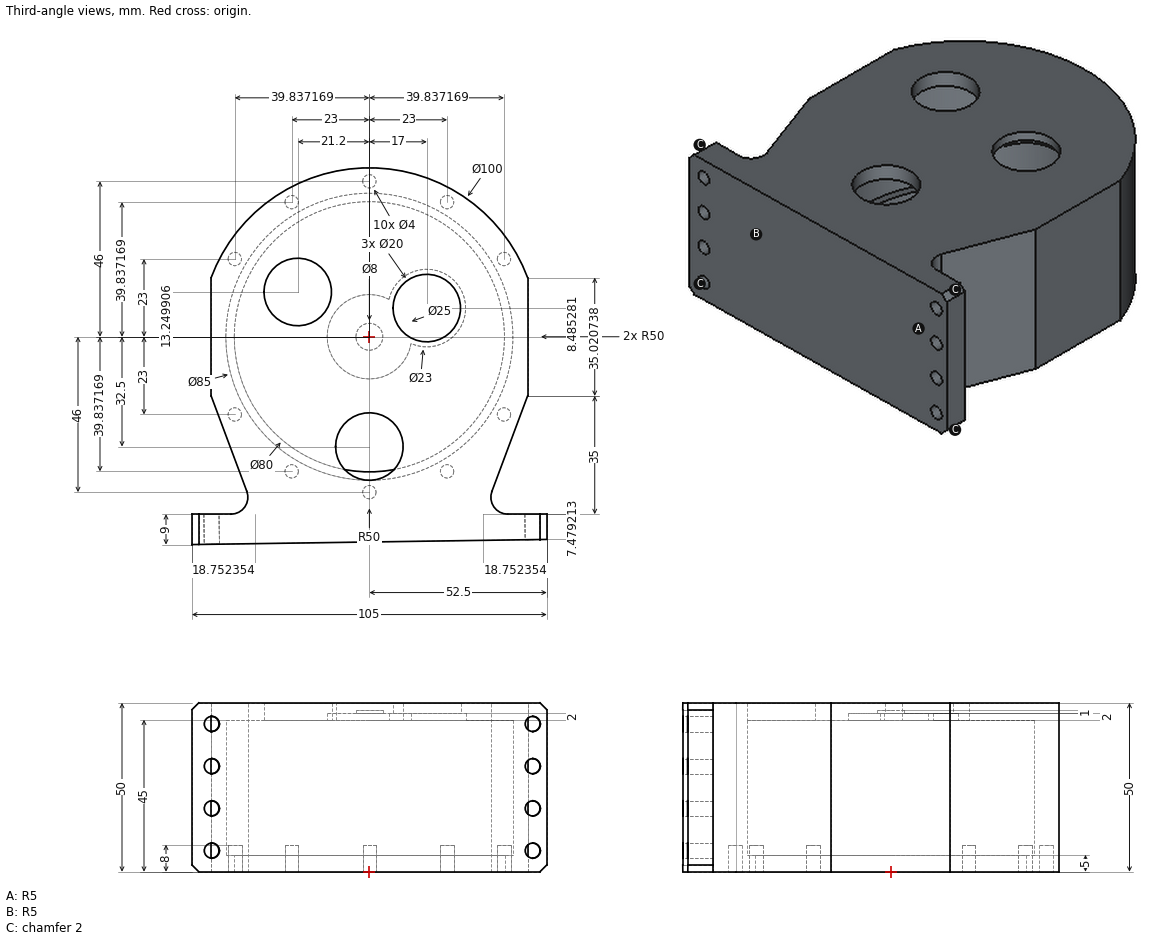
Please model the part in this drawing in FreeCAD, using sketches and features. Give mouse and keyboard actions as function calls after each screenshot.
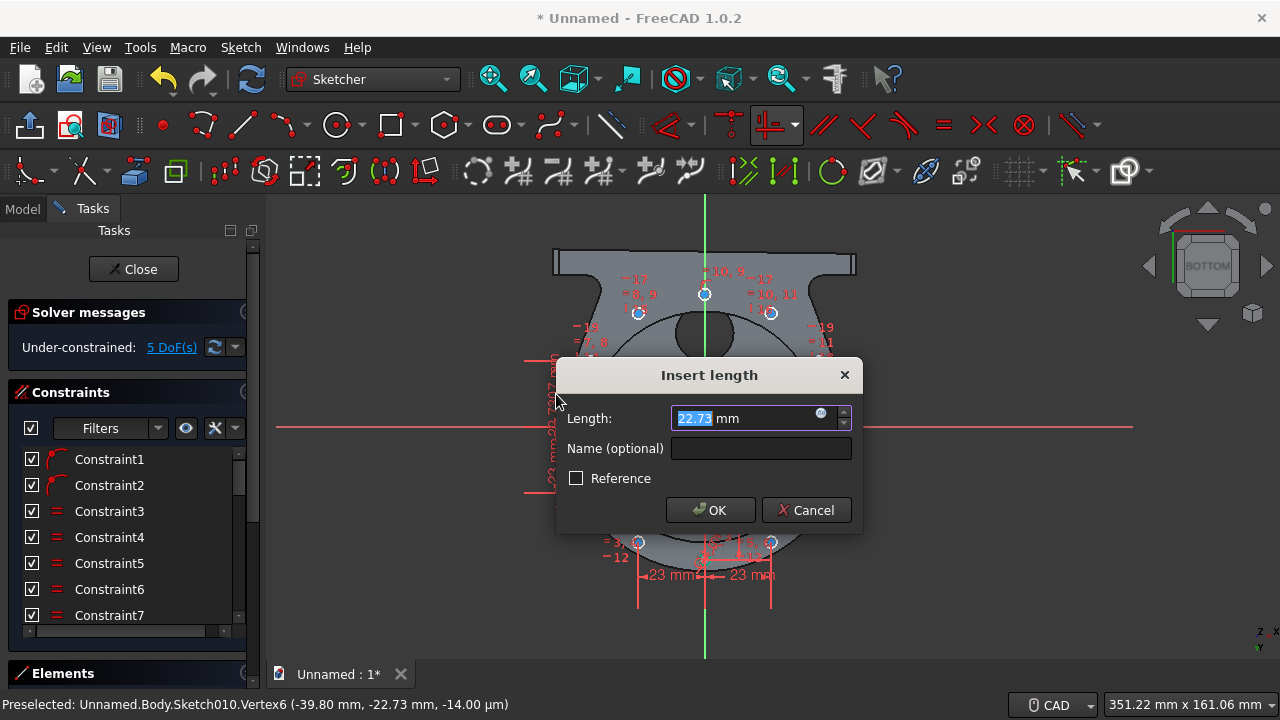
text(23)
key(Return)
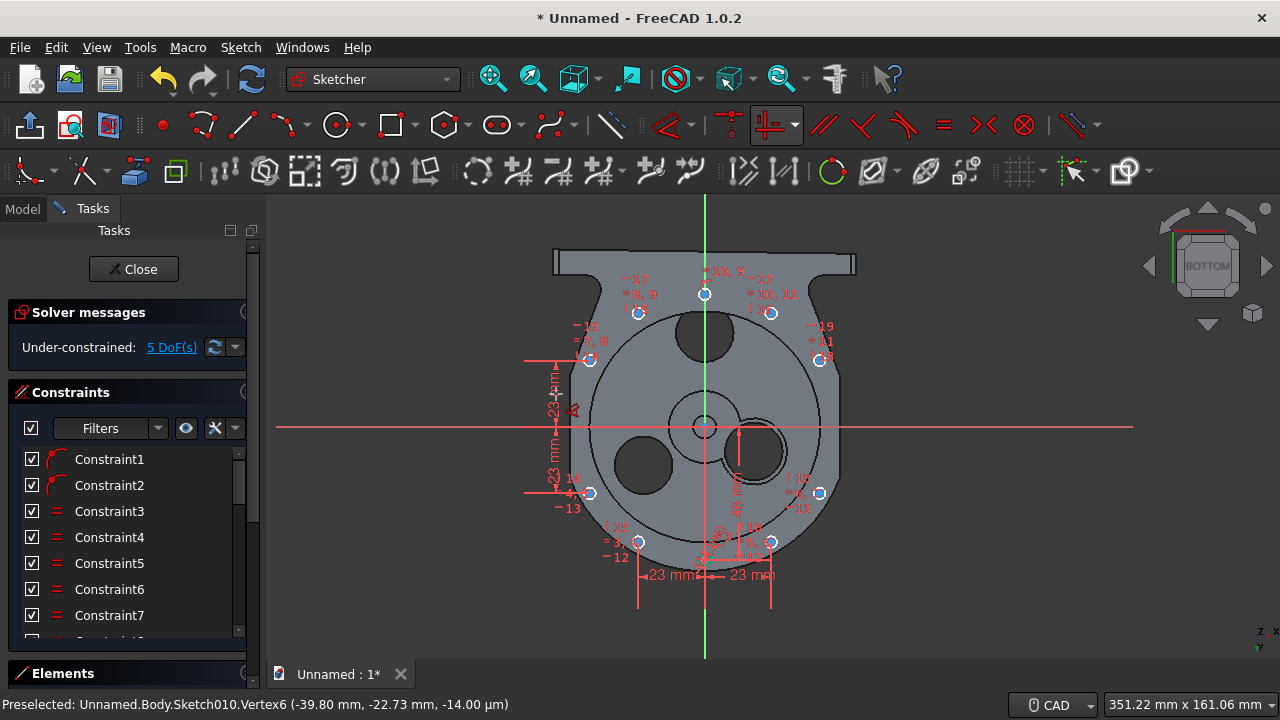
click(705, 294)
click(739, 361)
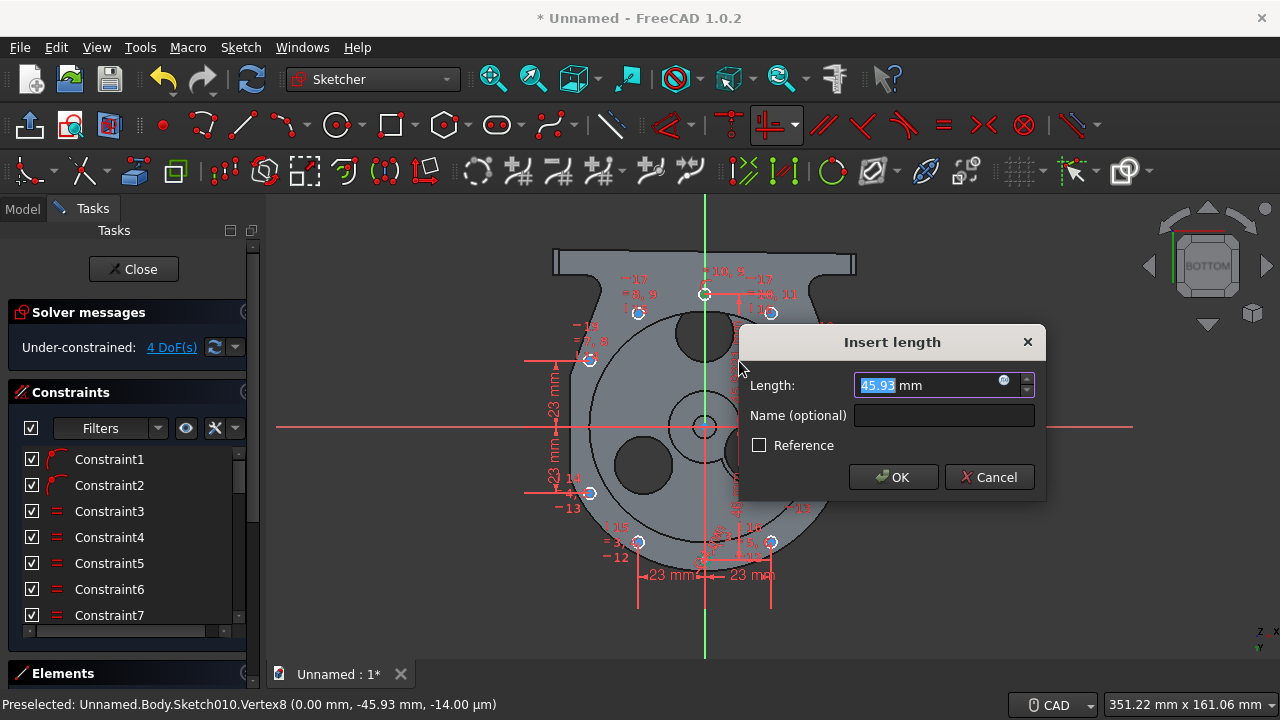
text(46)
key(Return)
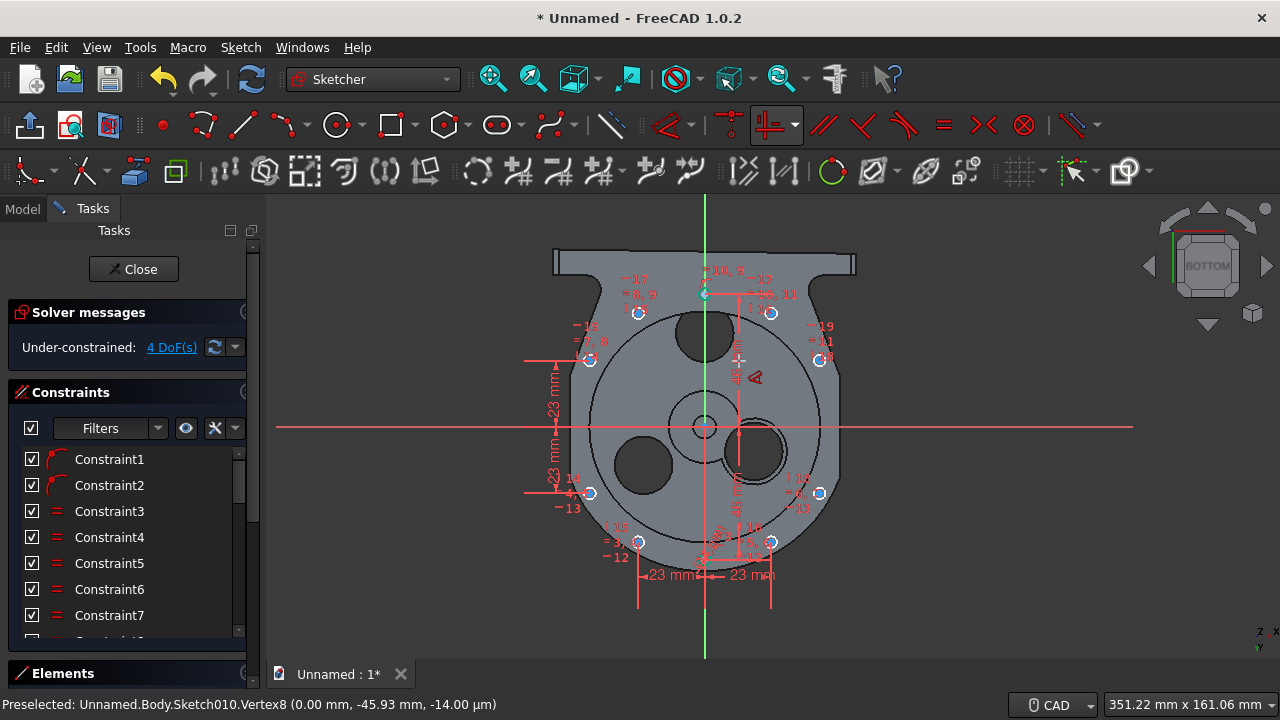
click(638, 542)
click(604, 511)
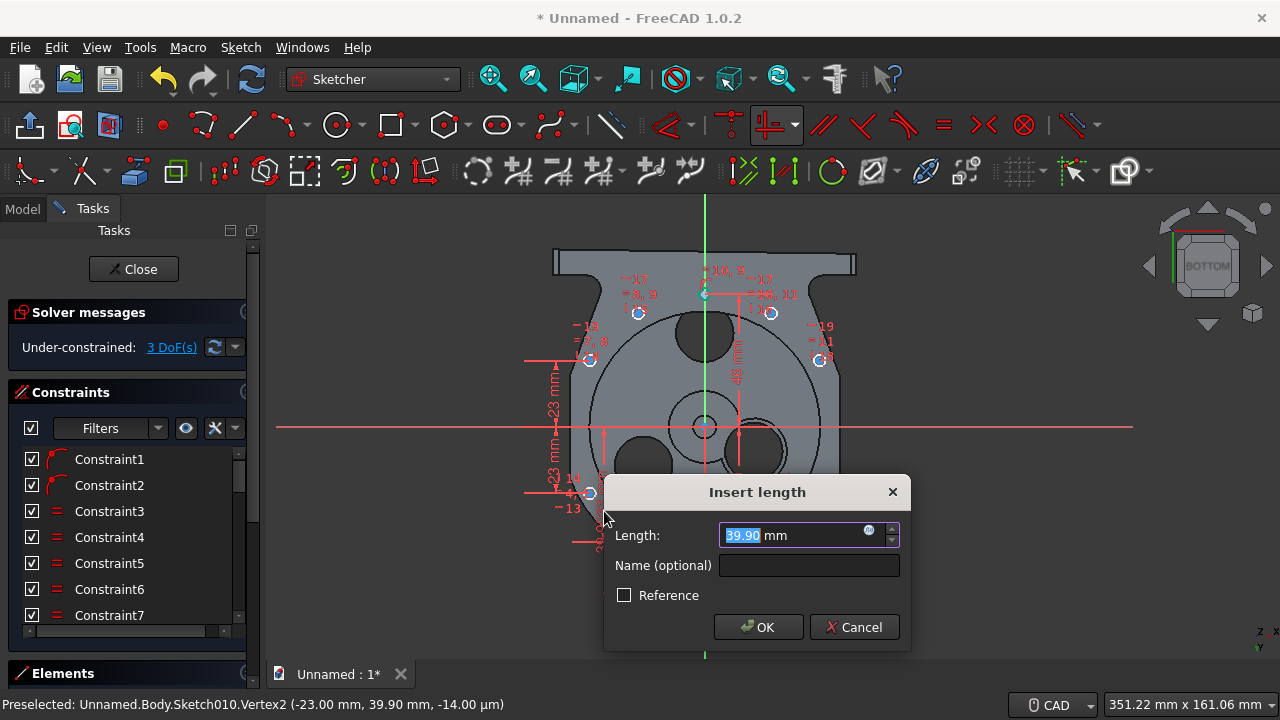
text(39.837169)
key(Return)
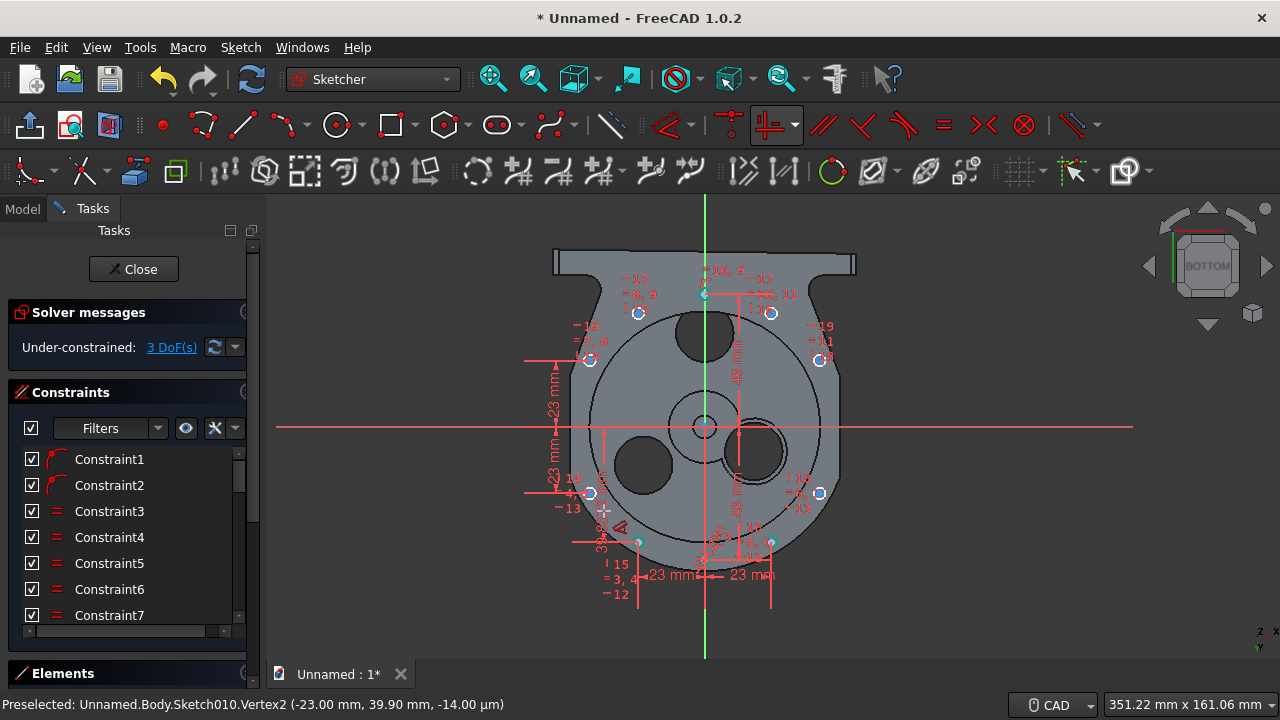
click(590, 493)
click(688, 527)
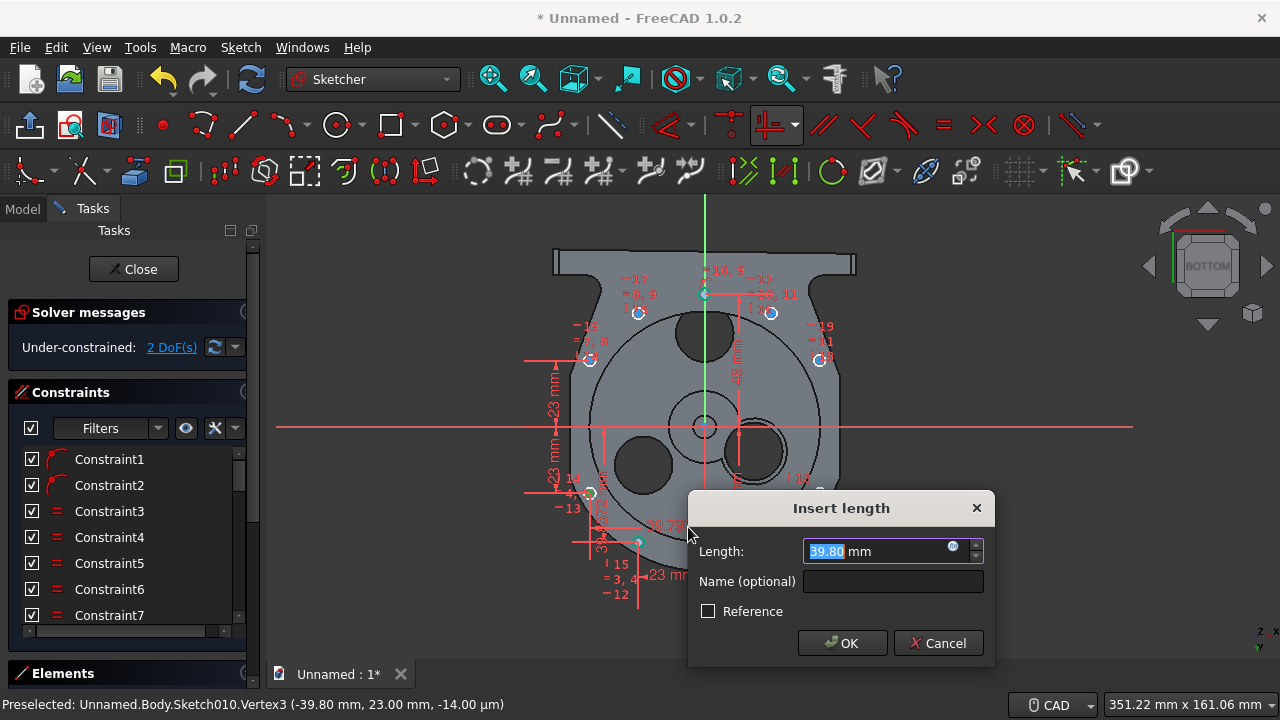
text(39.837169)
key(Return)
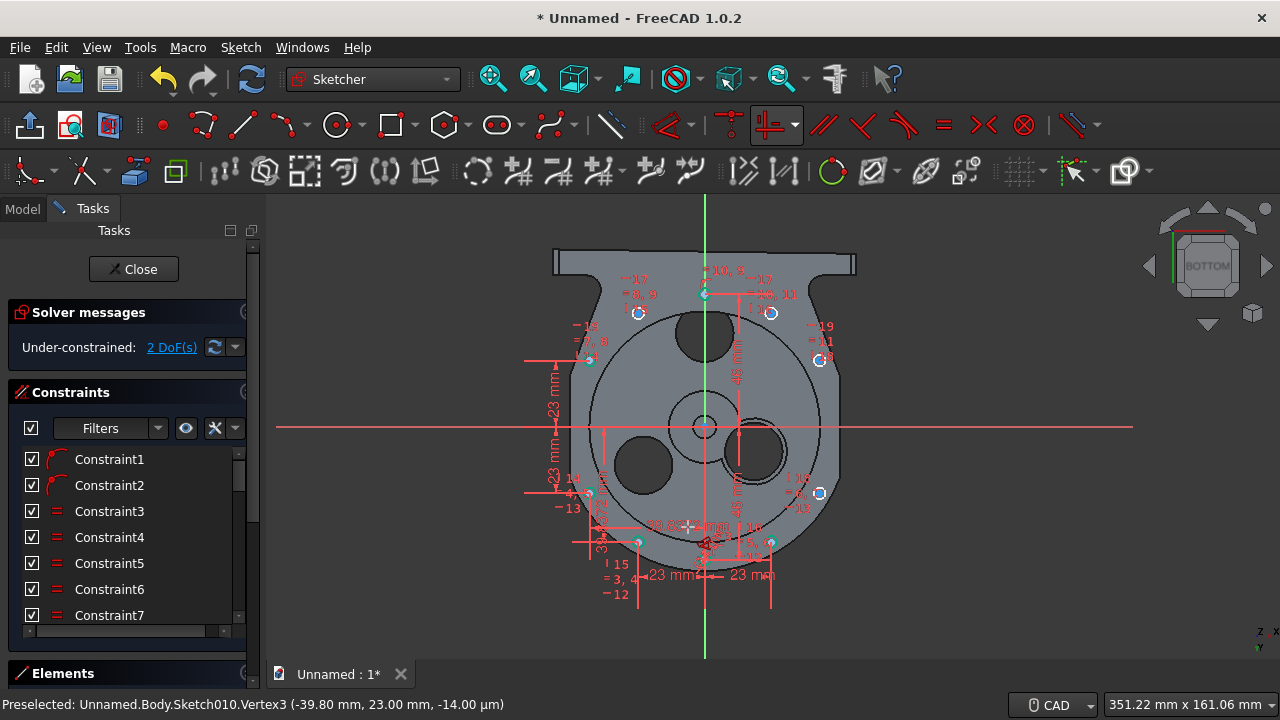
click(820, 493)
click(789, 527)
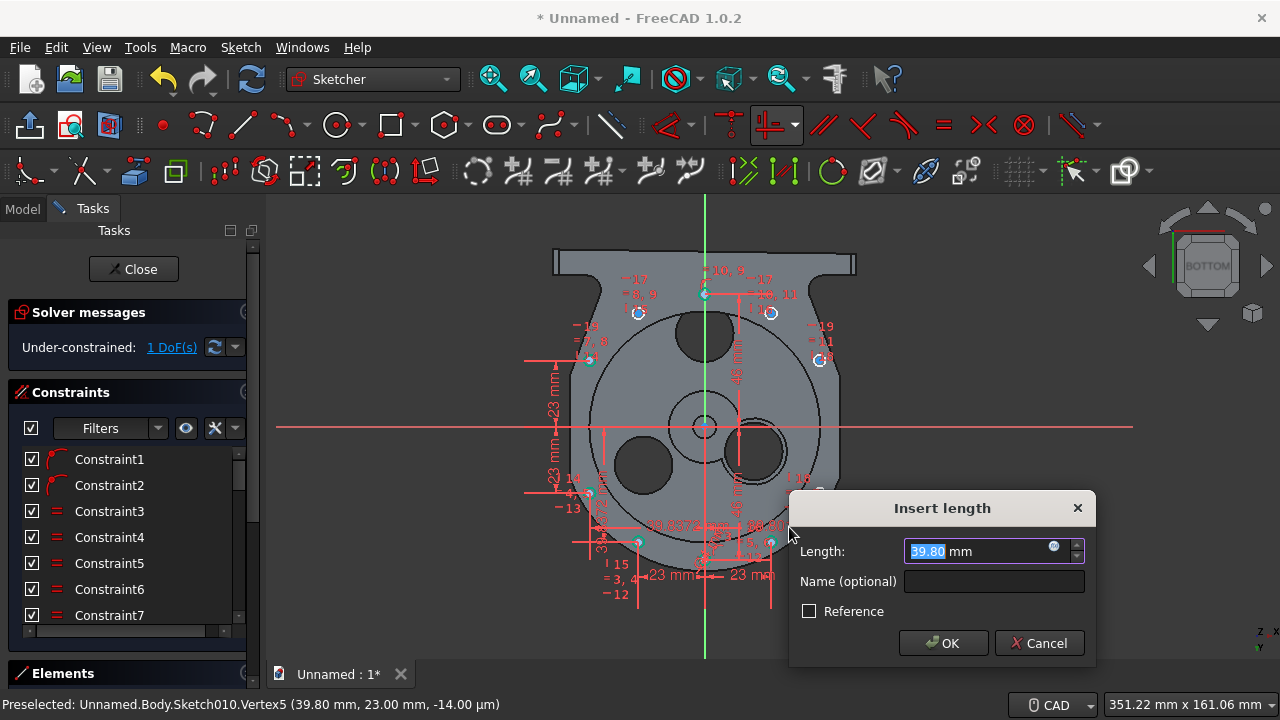
text(39.837169)
key(Return)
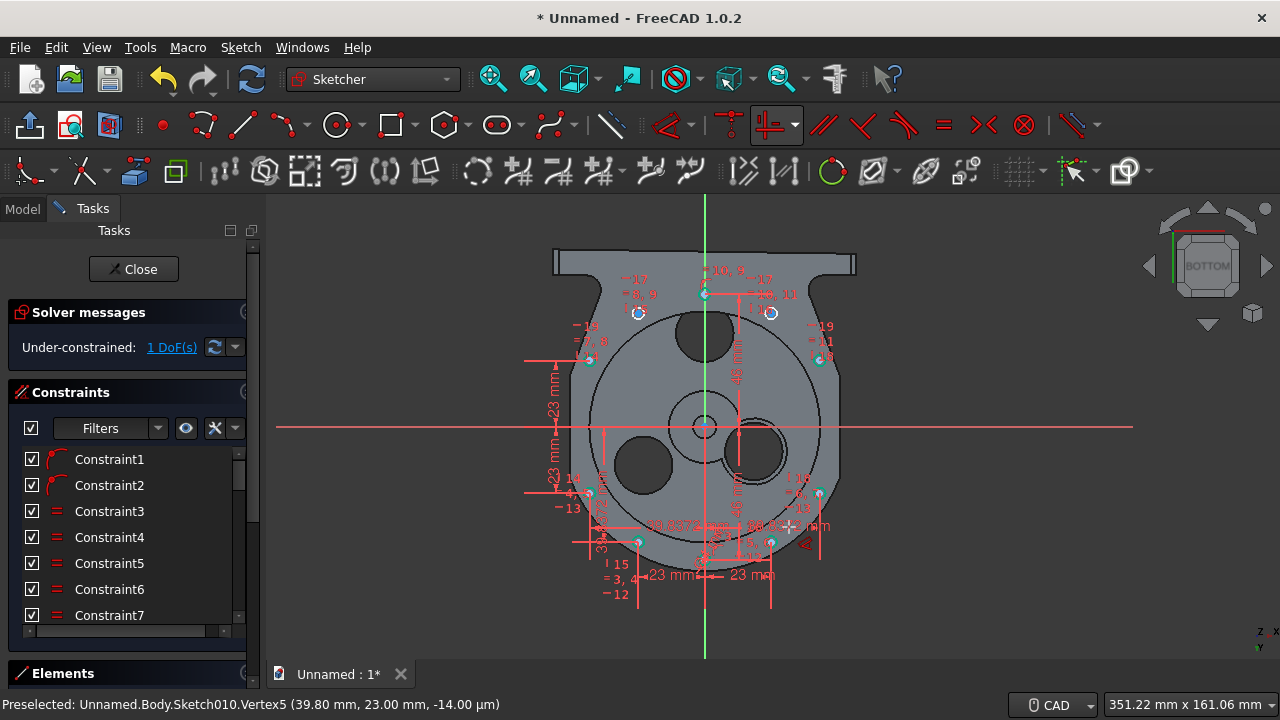
click(638, 313)
click(604, 344)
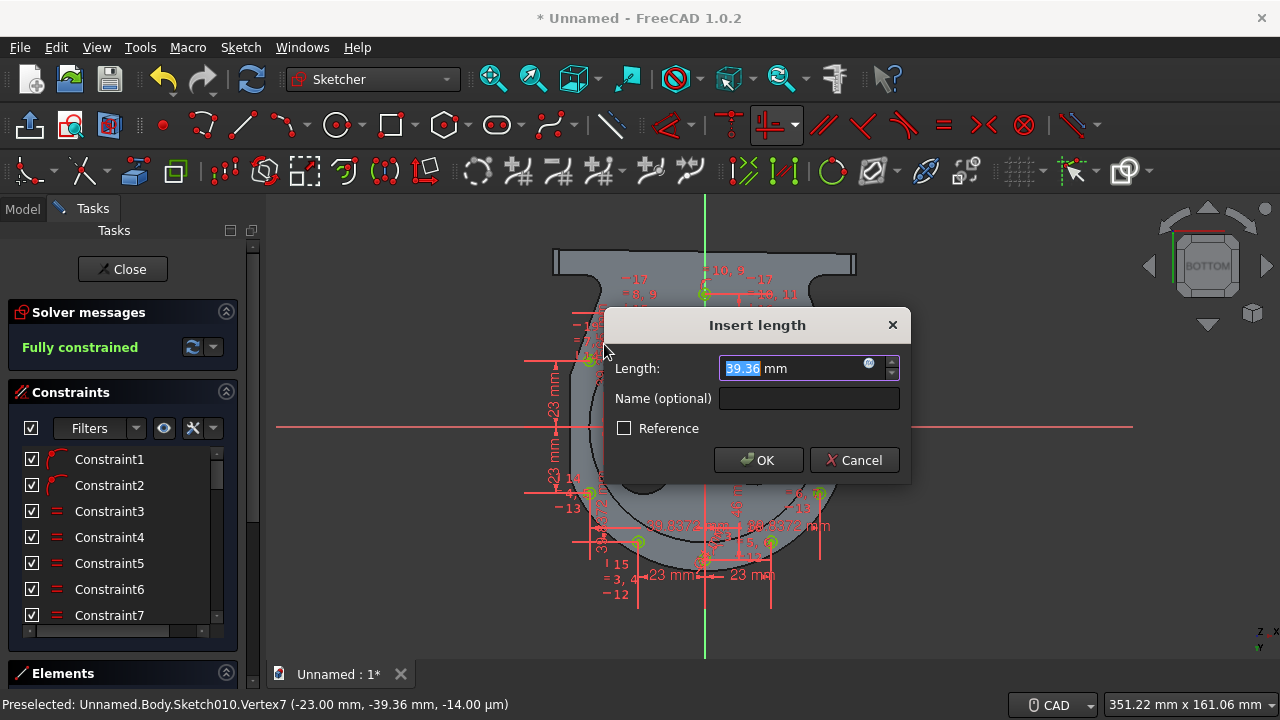
text(39.837169)
key(Return)
key(Escape)